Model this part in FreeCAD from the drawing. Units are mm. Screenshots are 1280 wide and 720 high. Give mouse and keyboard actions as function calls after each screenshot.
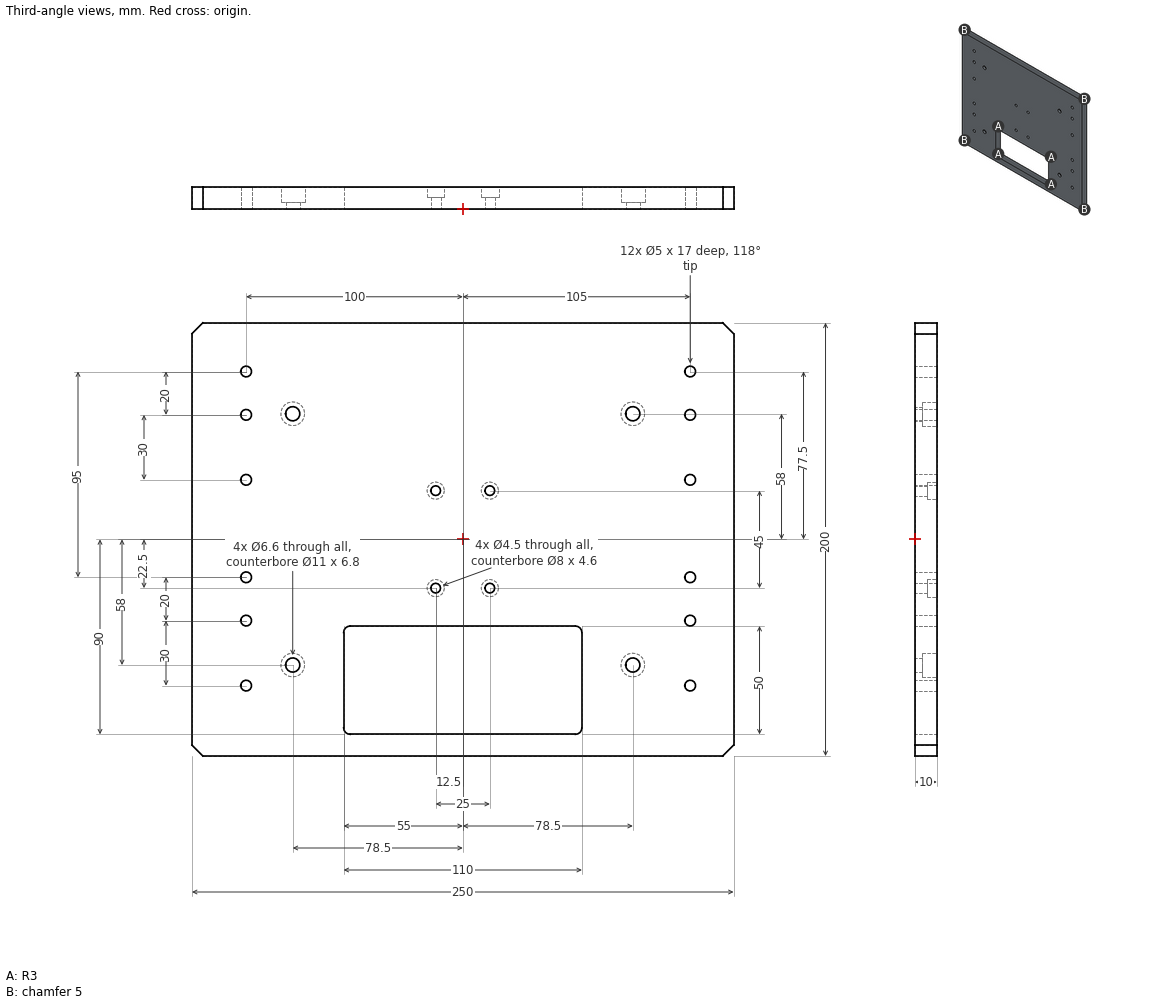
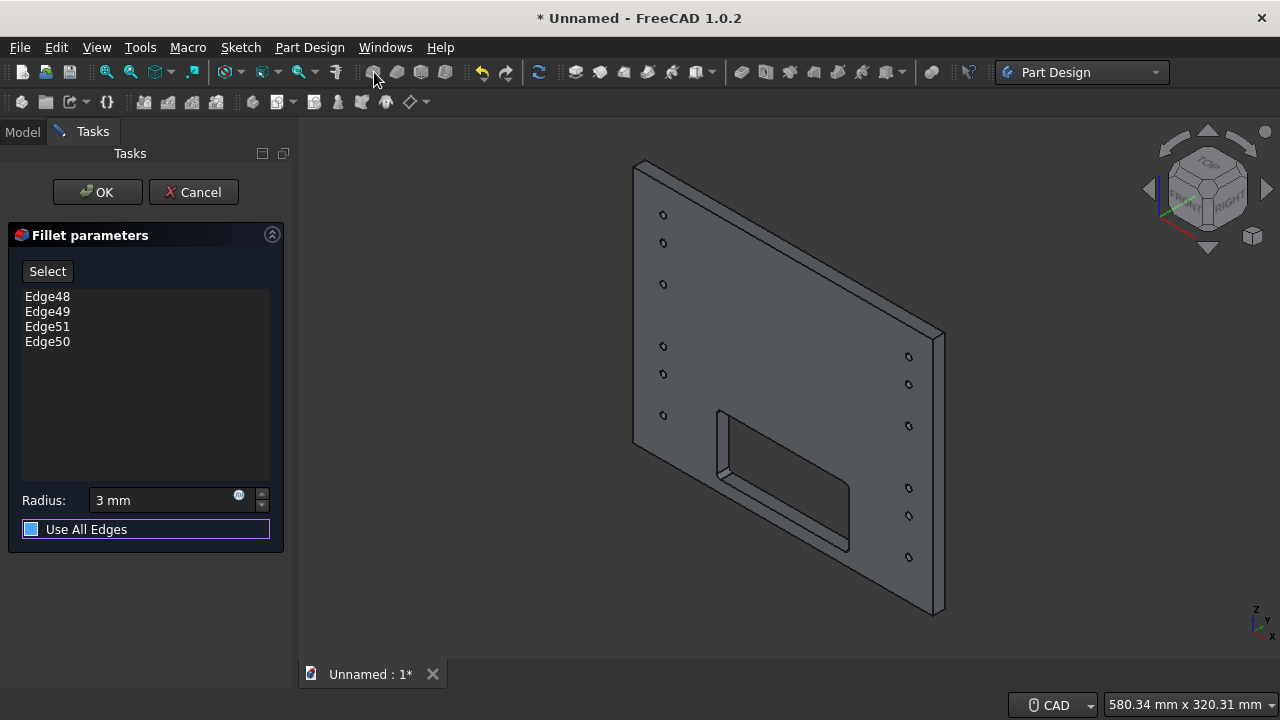
click(98, 192)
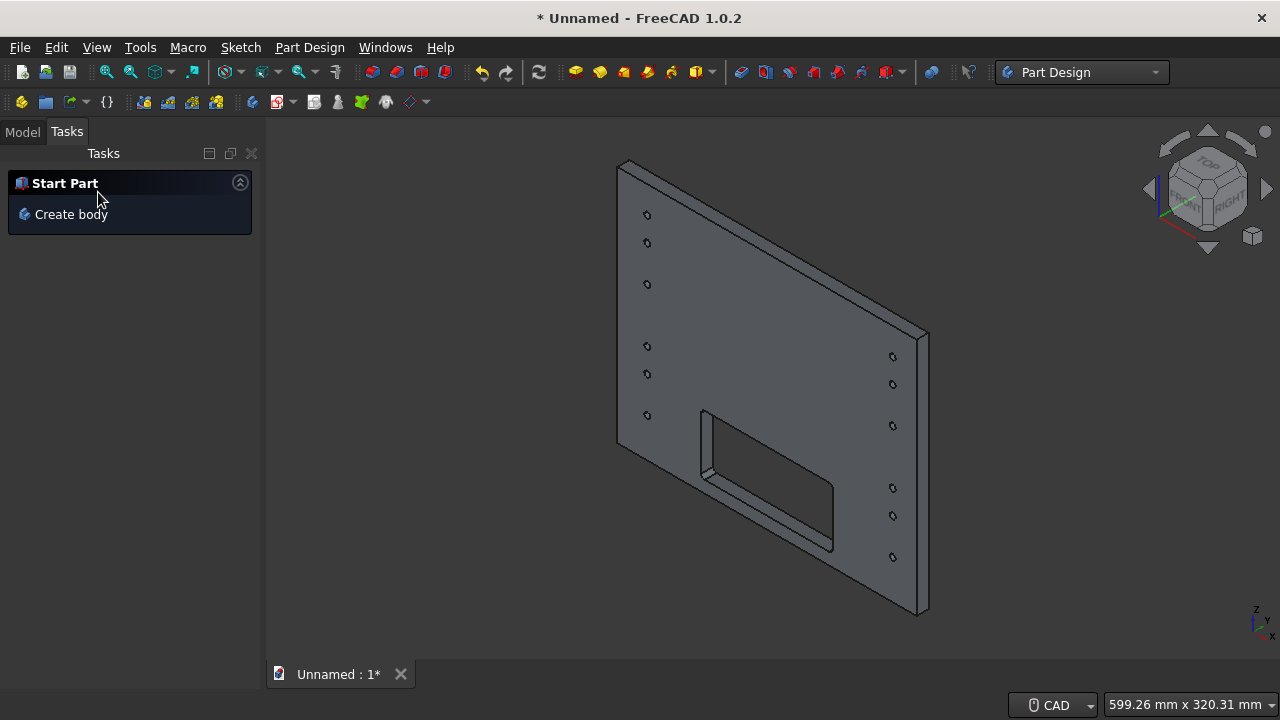
click(923, 335)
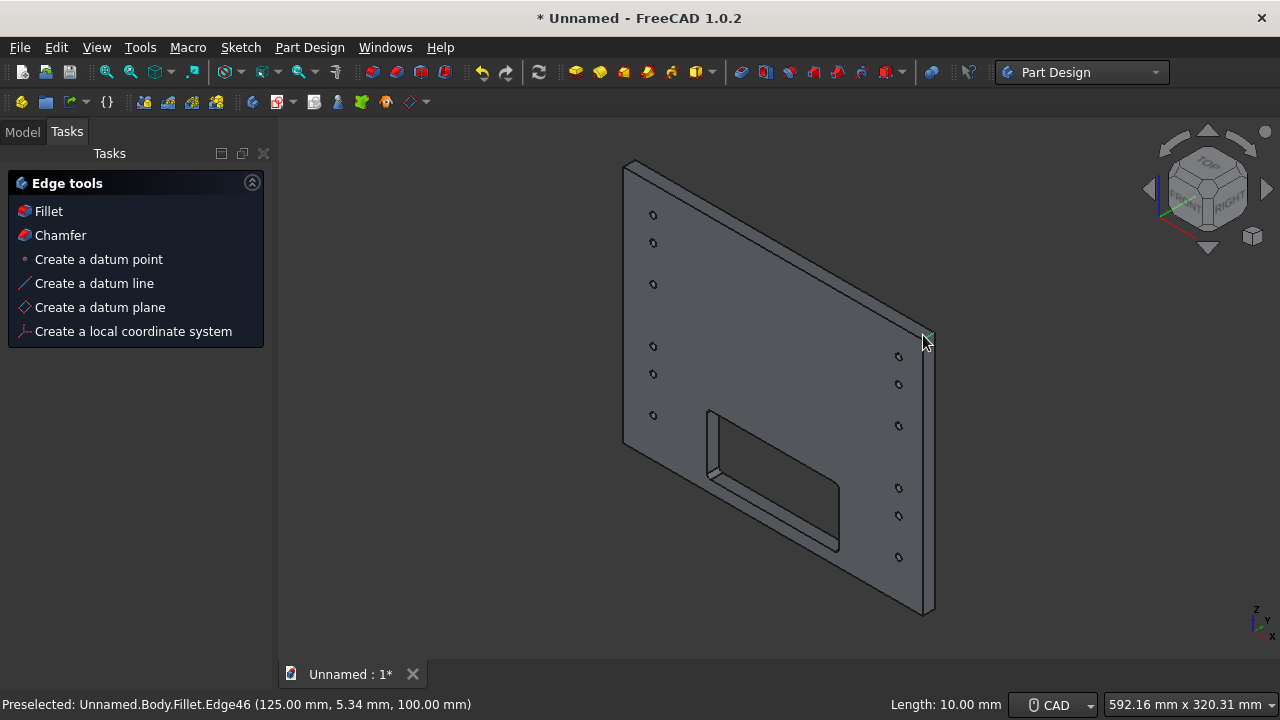
scroll(629, 162, up, 5)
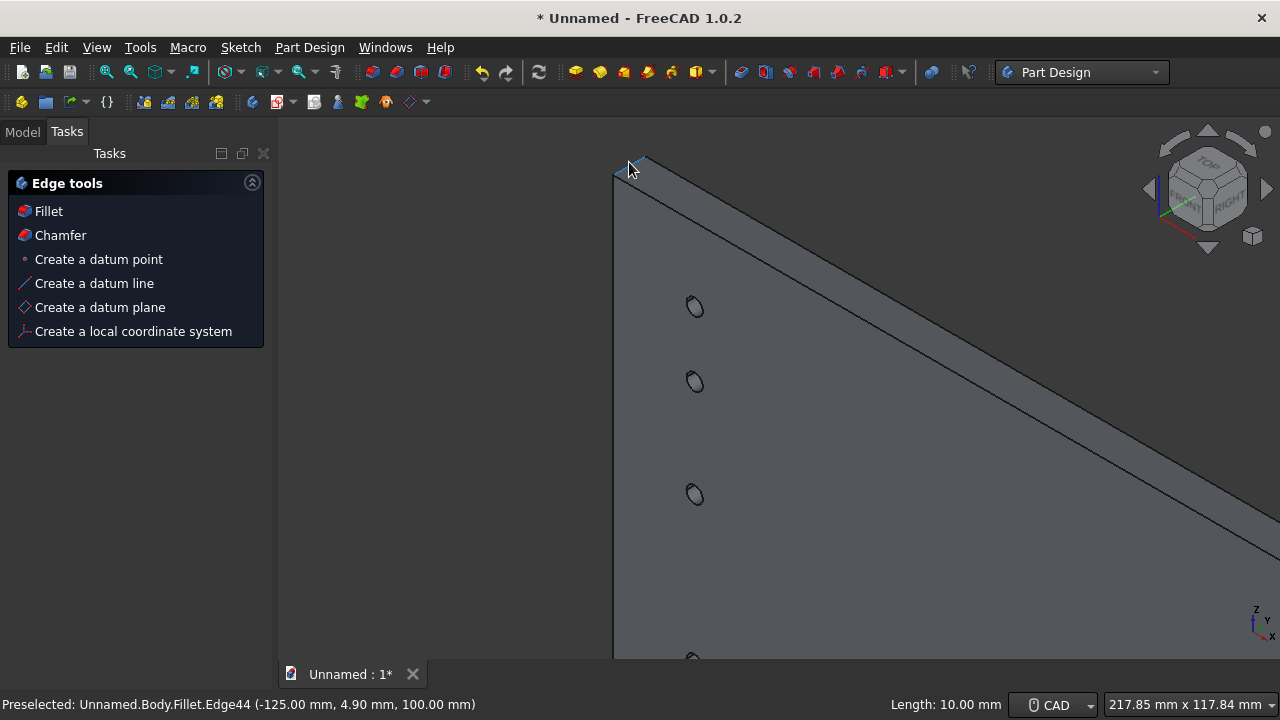
click(108, 72)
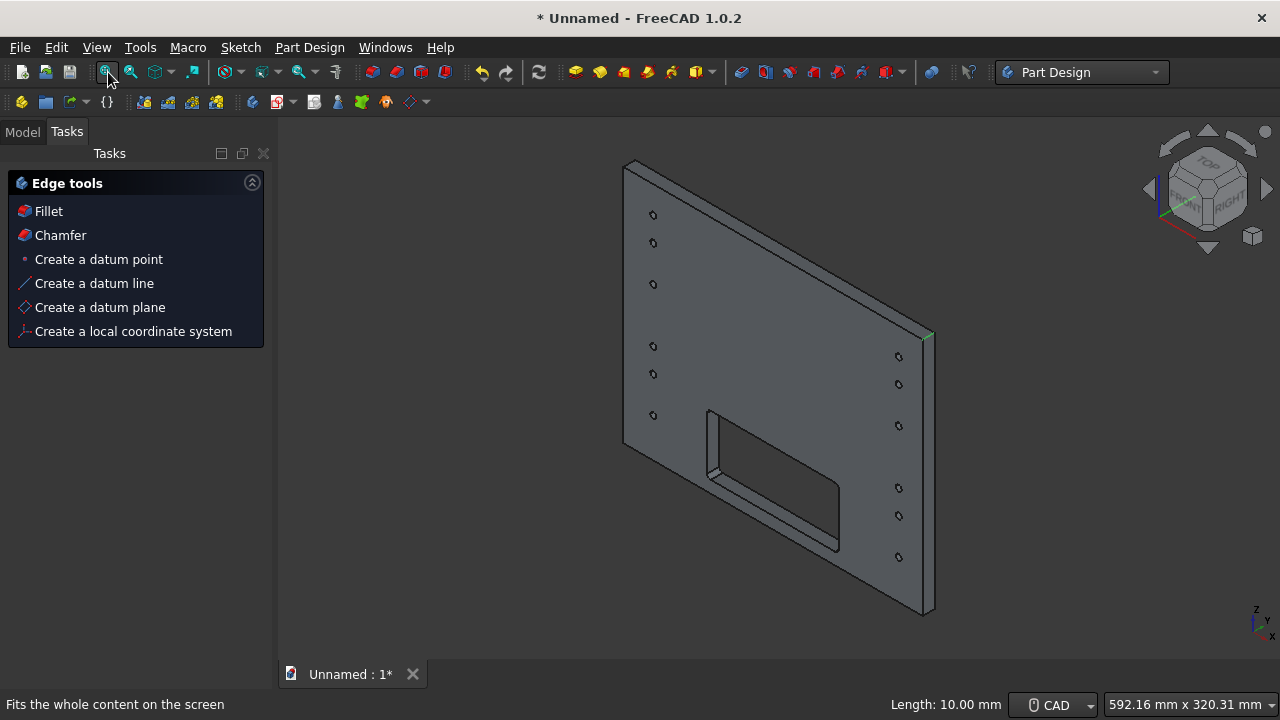
key(2)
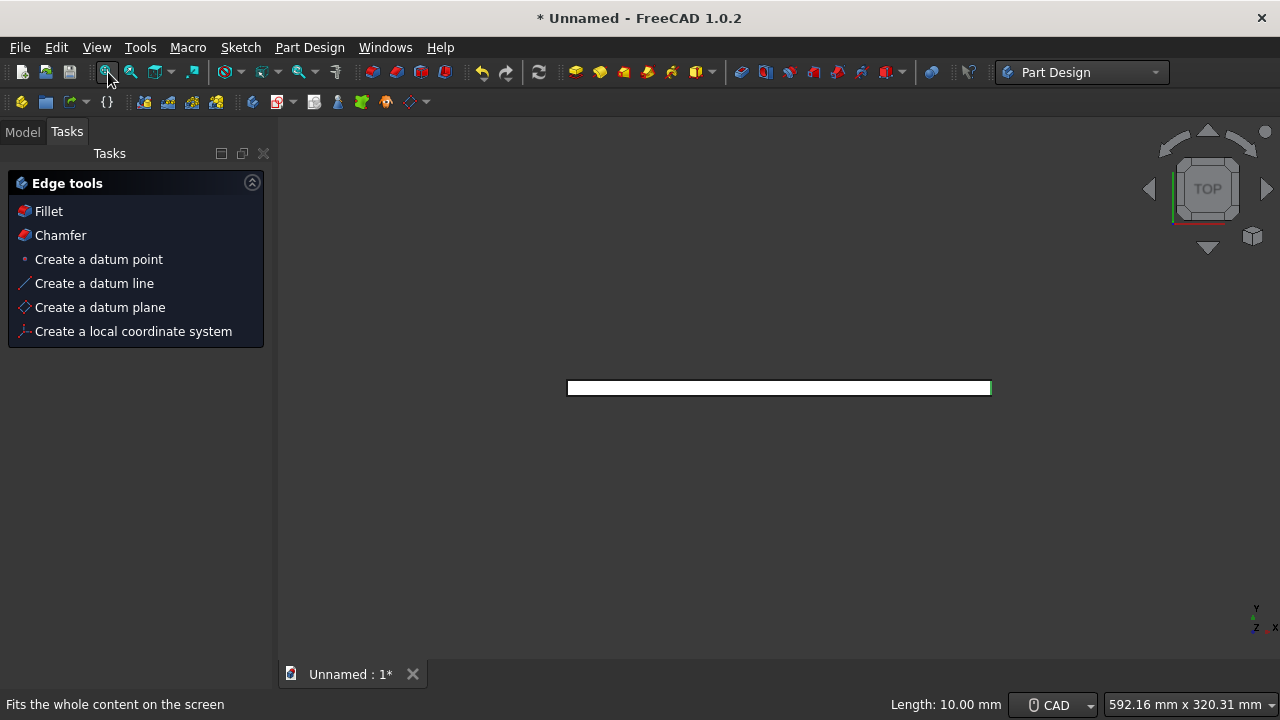
click(108, 72)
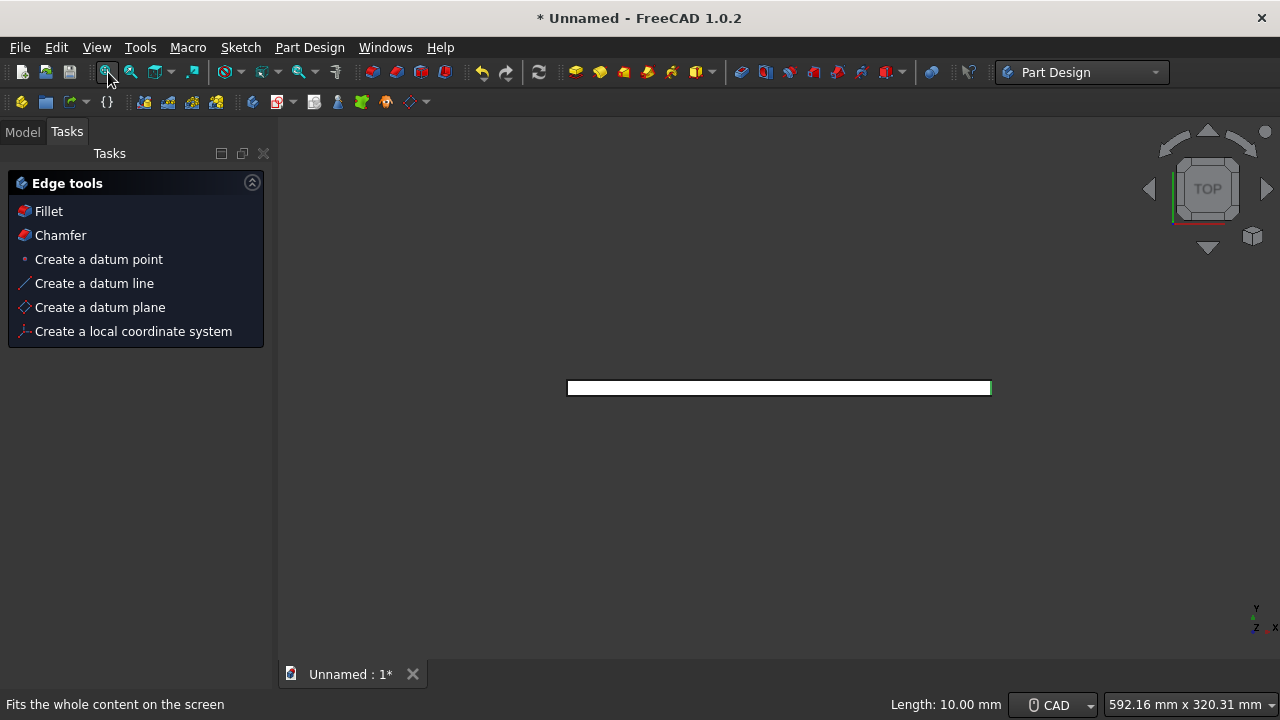
click(567, 387, ctrl)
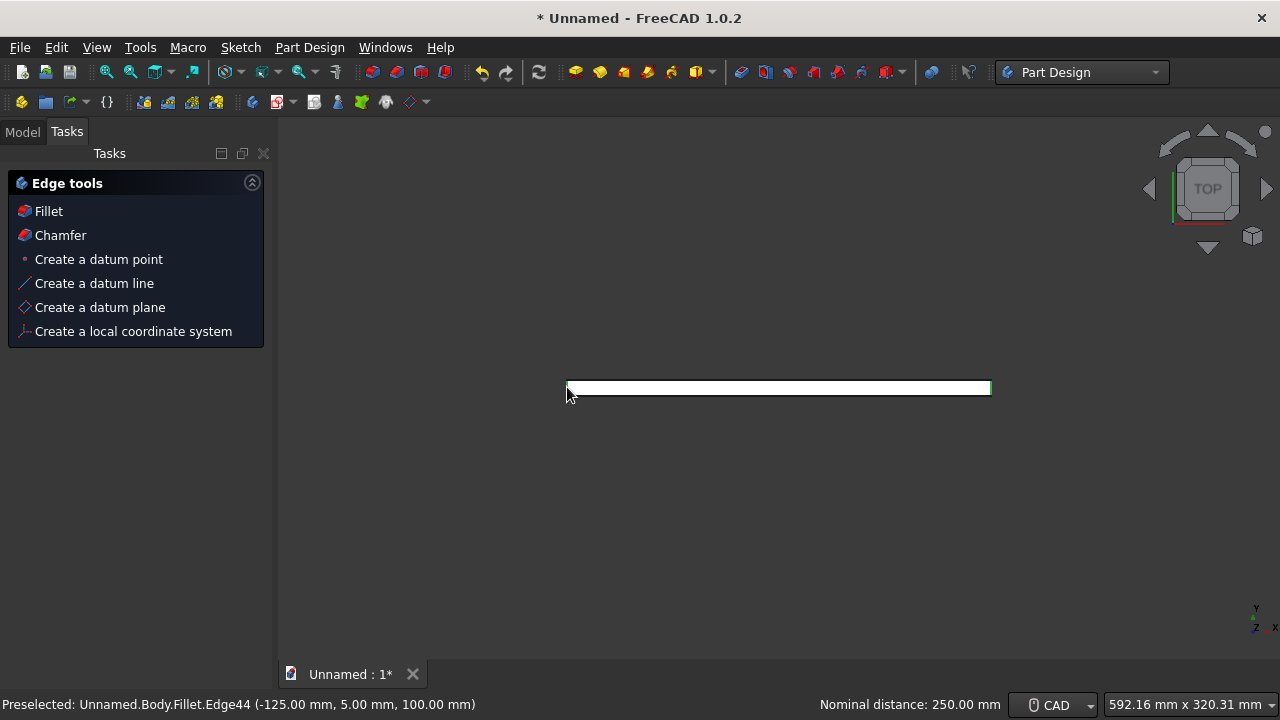
scroll(567, 387, up, 5)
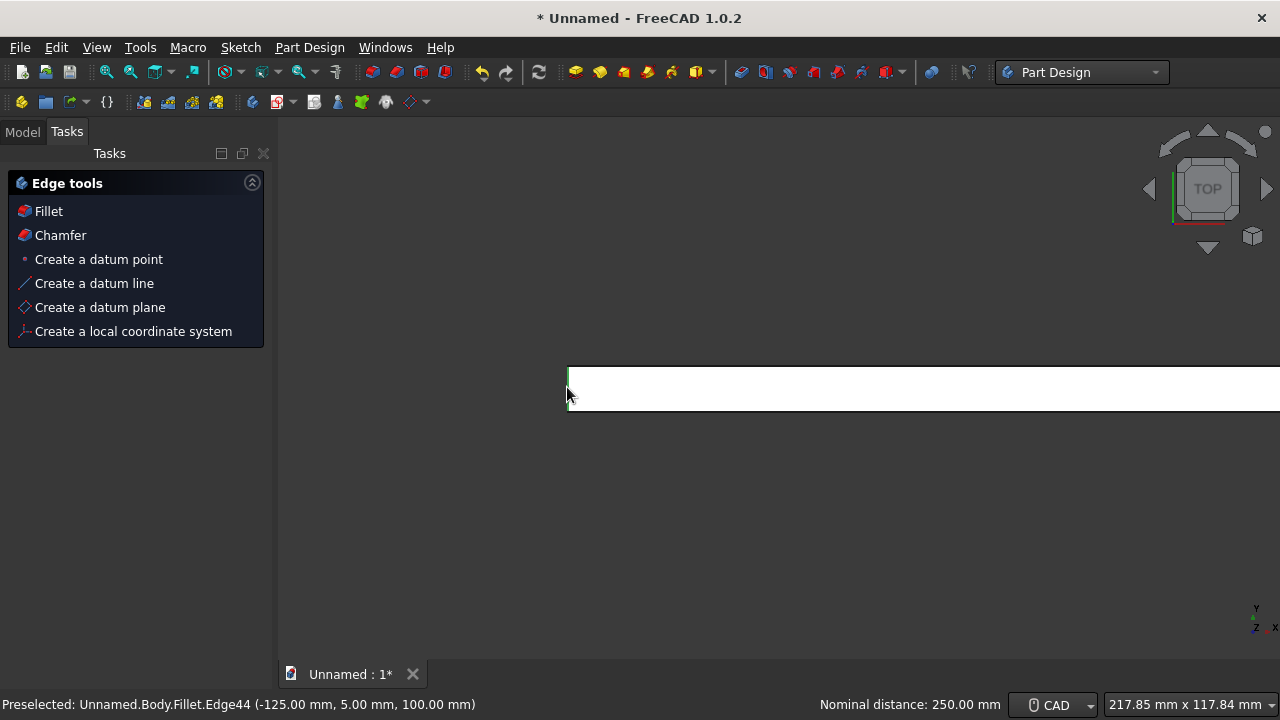
click(108, 72)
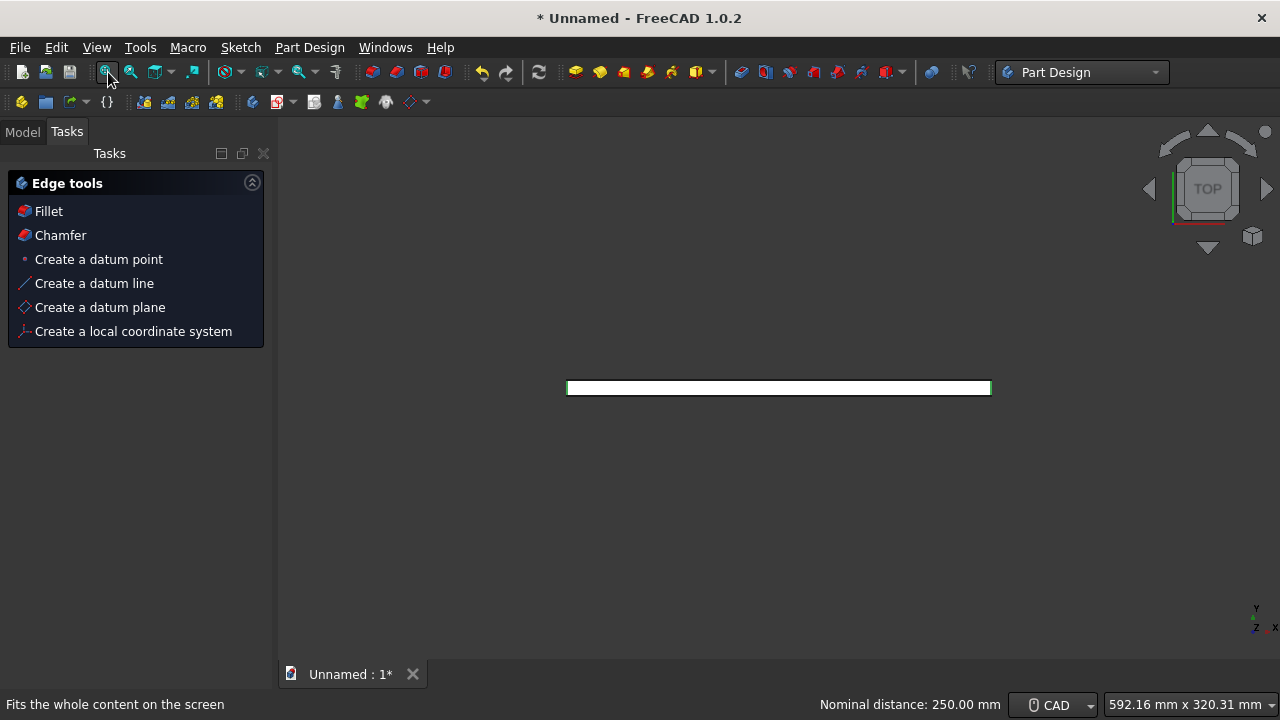
key(0)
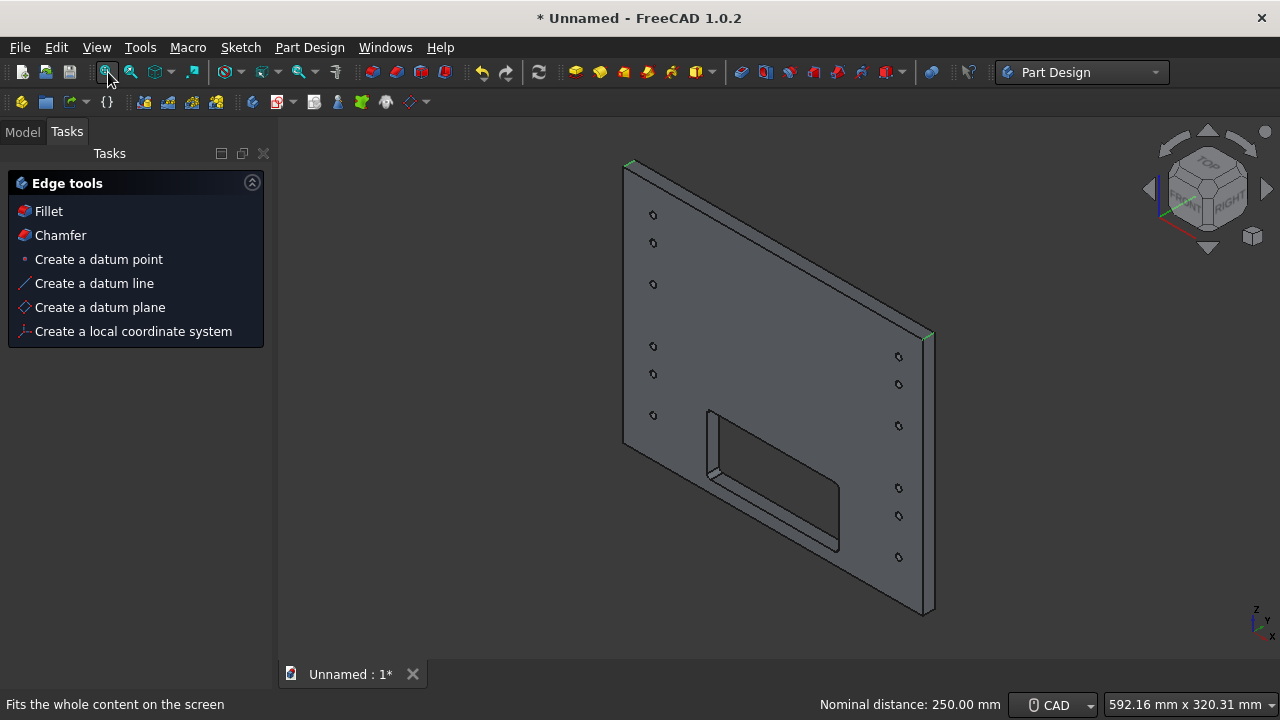
scroll(629, 439, up, 5)